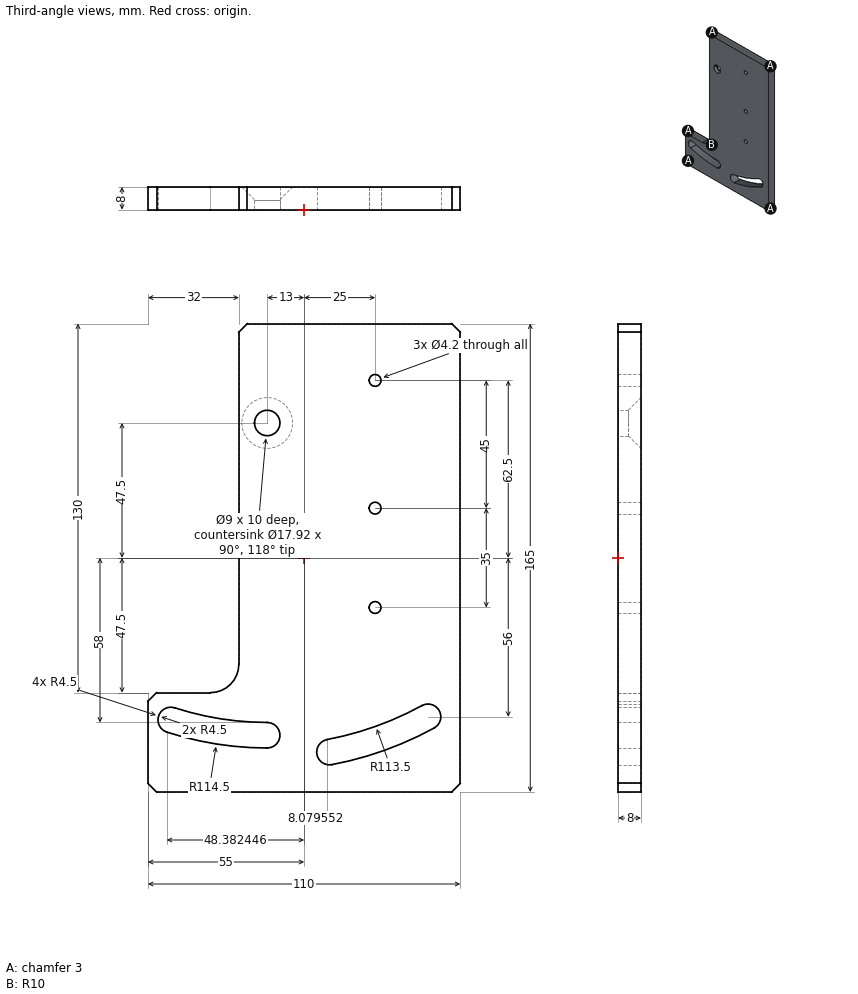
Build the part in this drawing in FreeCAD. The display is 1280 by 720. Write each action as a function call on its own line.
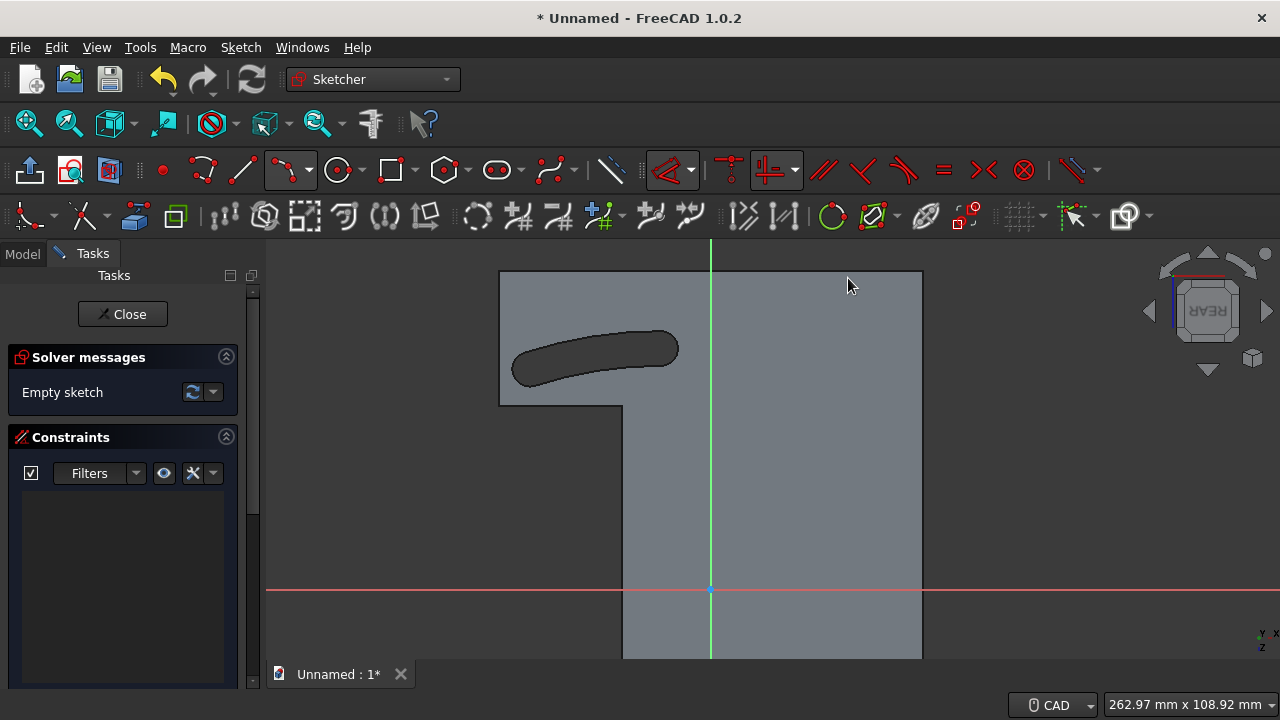
click(284, 170)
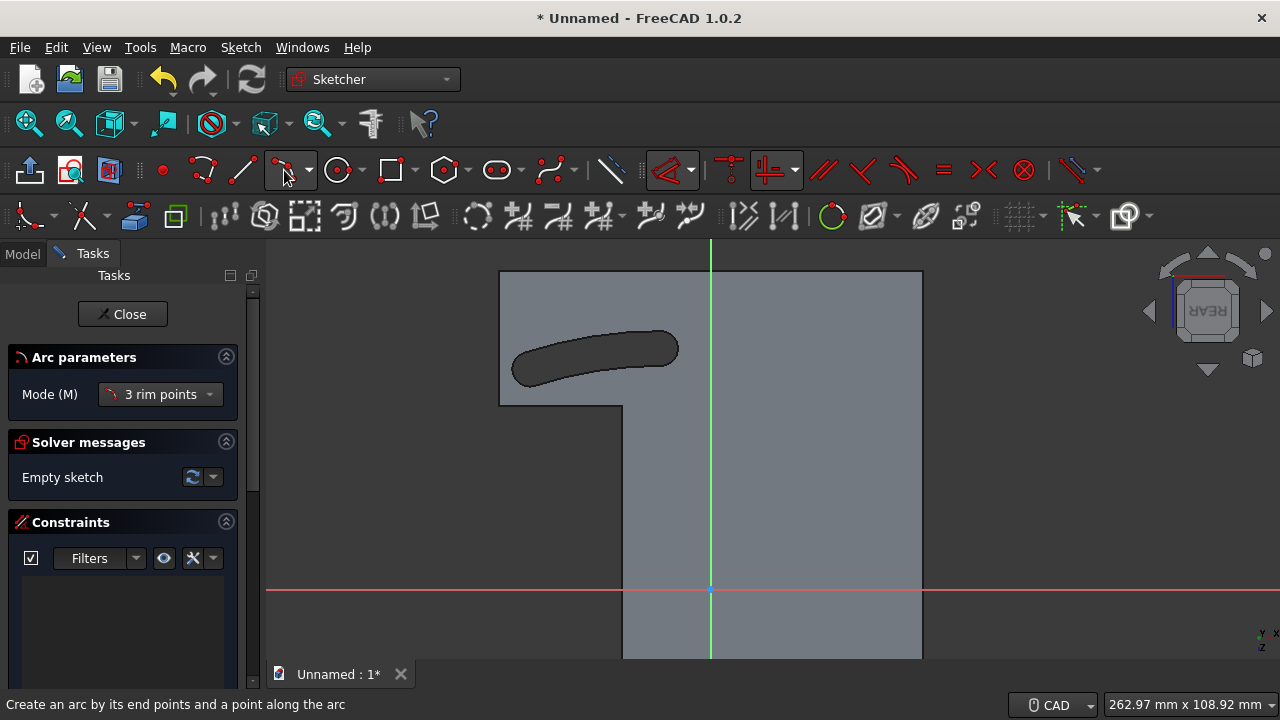
click(661, 366)
click(661, 331)
click(678, 349)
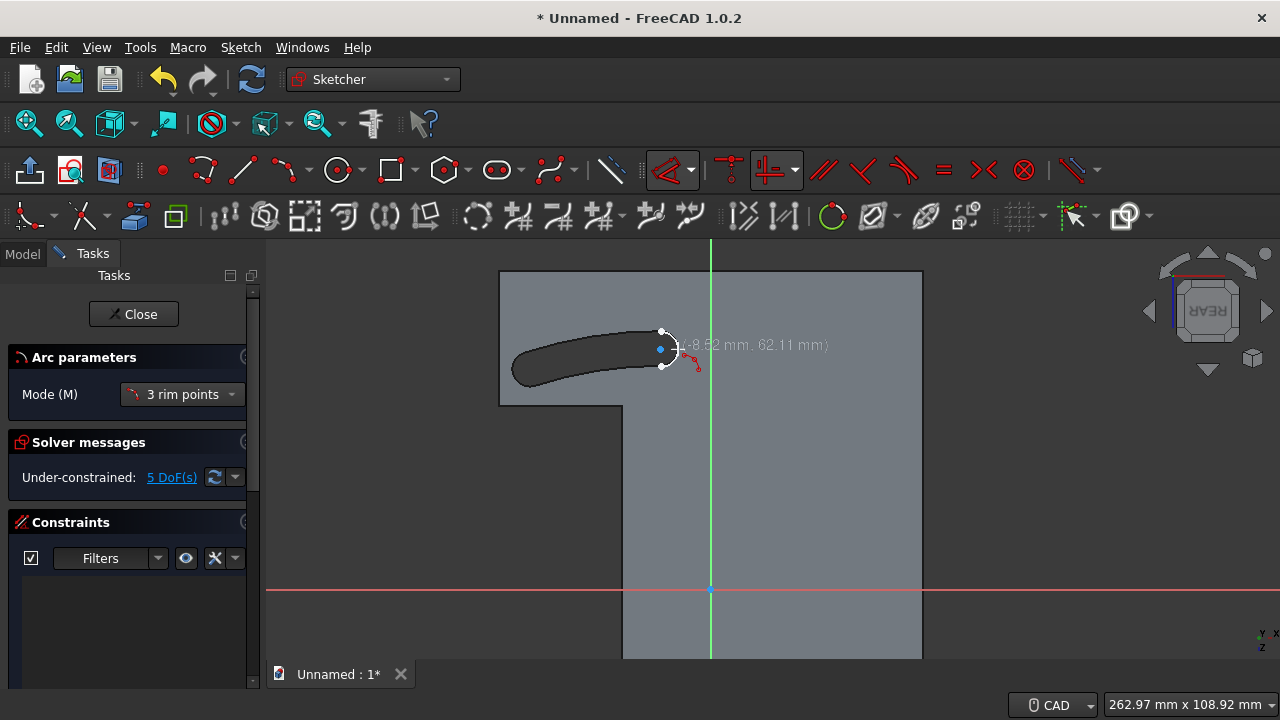
click(661, 332)
click(524, 353)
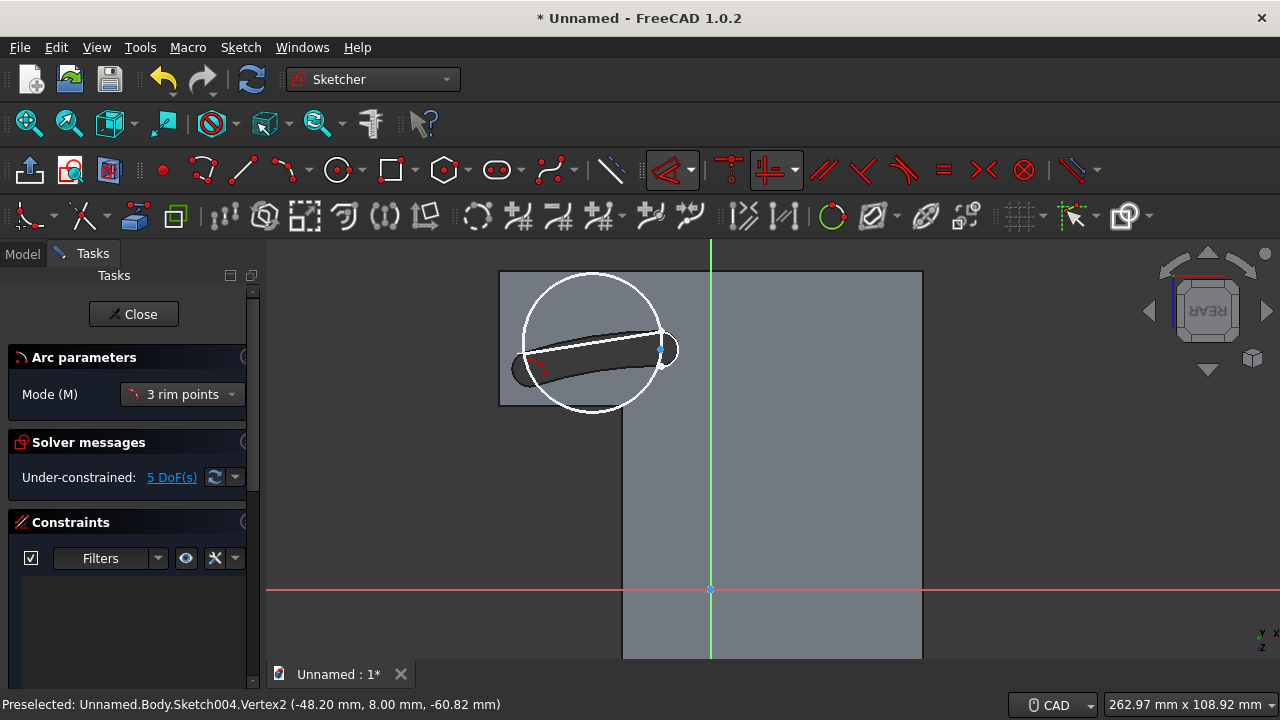
scroll(592, 337, up, 6)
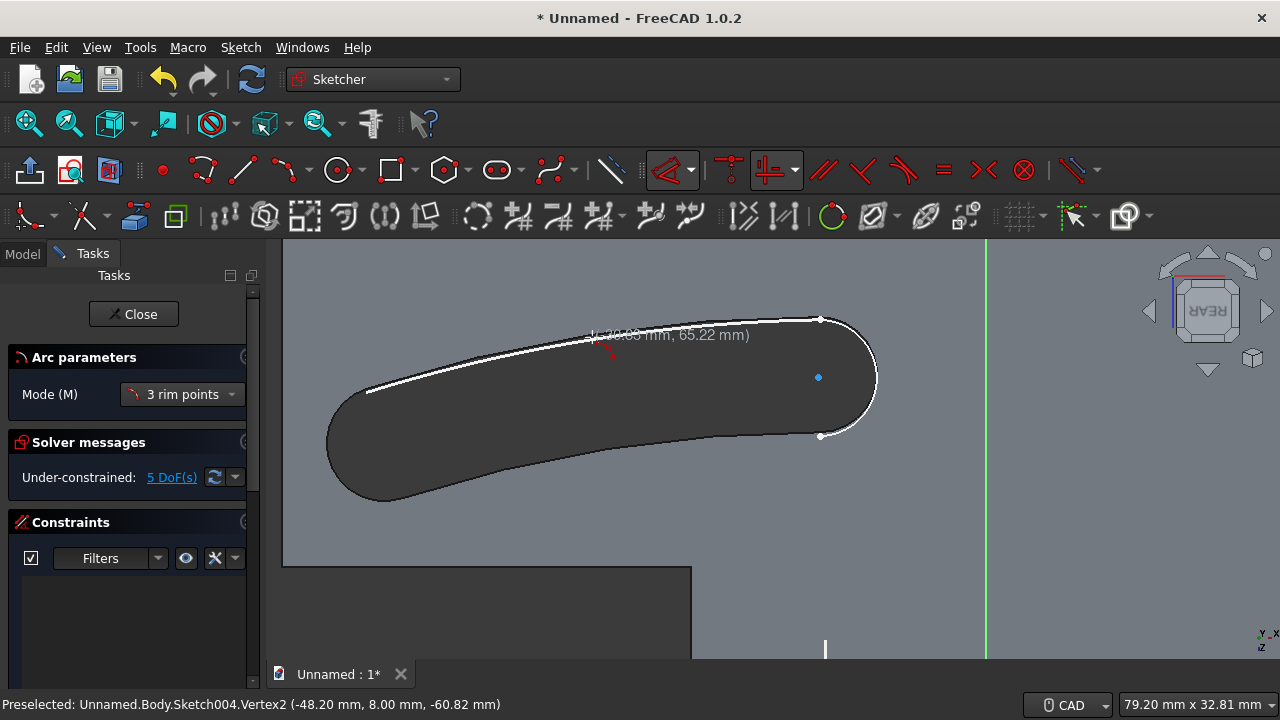
click(590, 335)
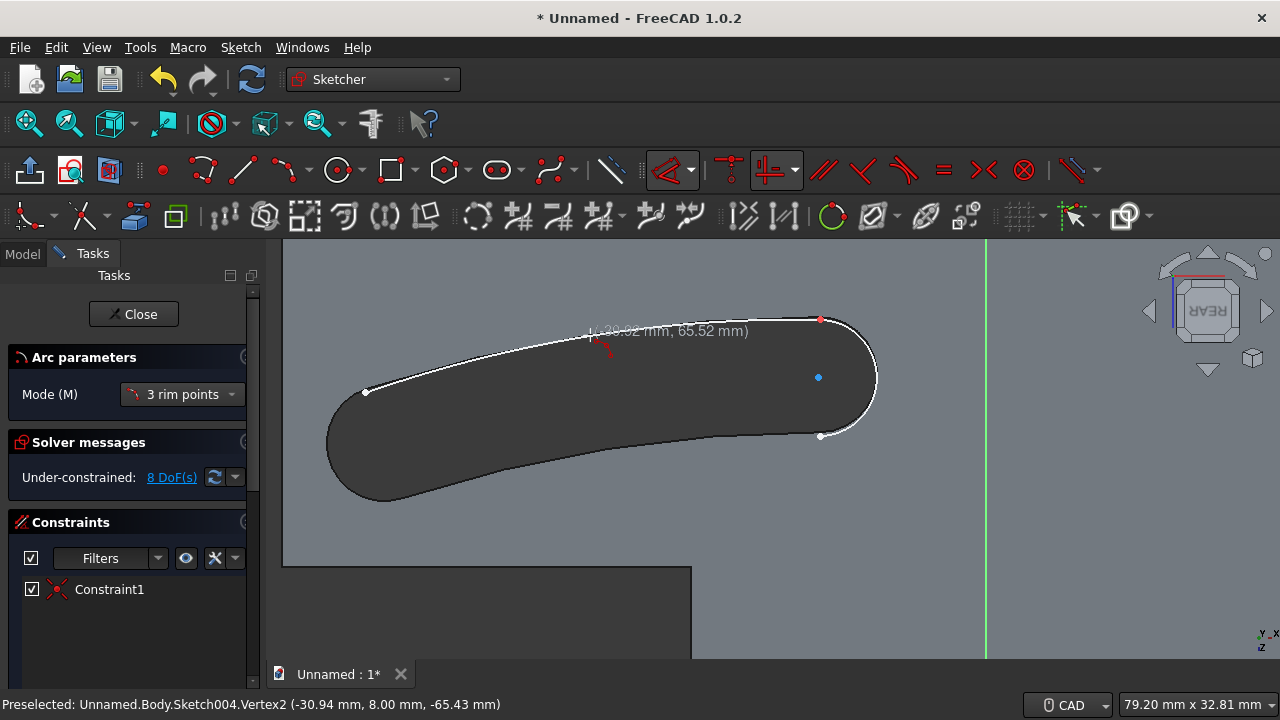
click(365, 393)
click(402, 498)
click(330, 461)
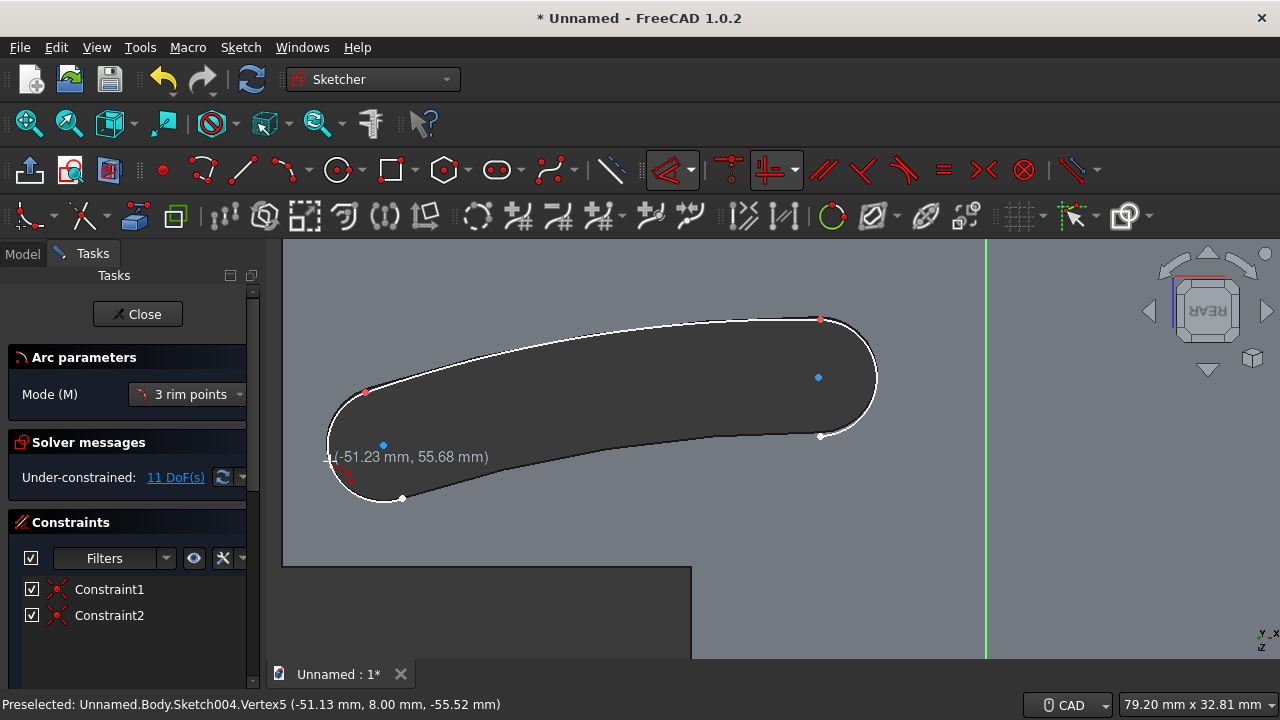
click(402, 499)
click(820, 436)
click(608, 449)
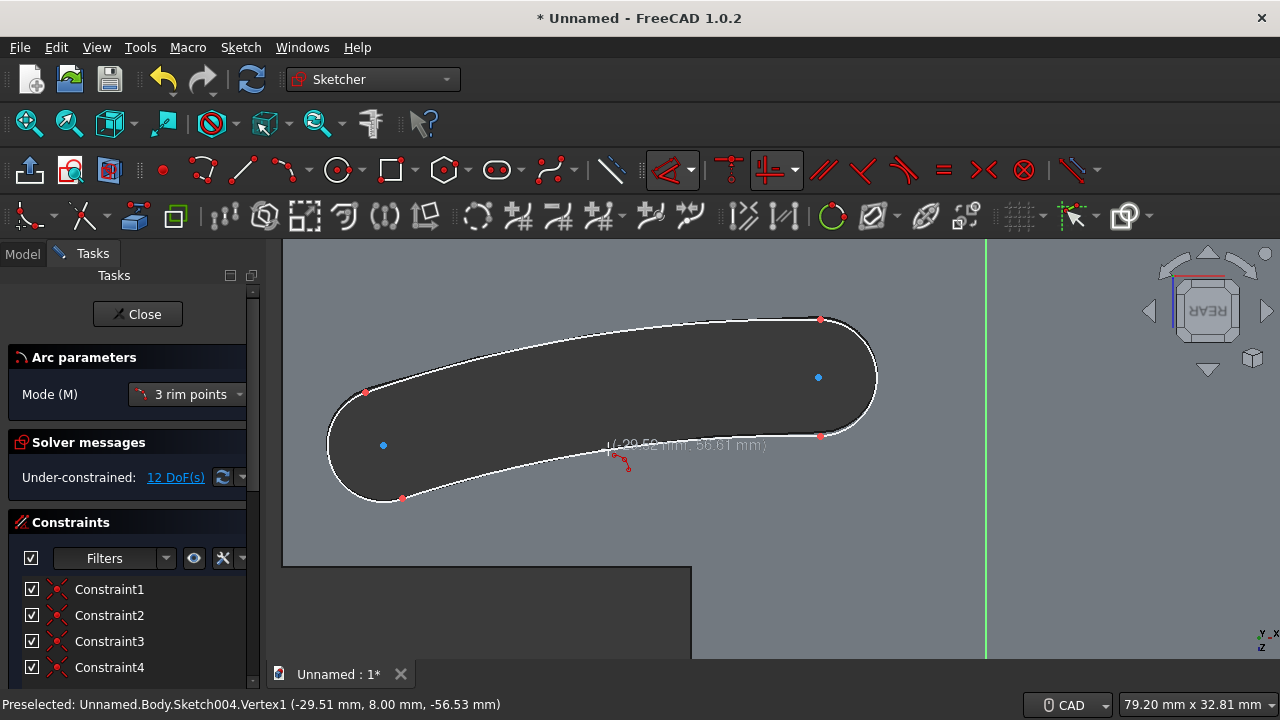
click(1089, 355)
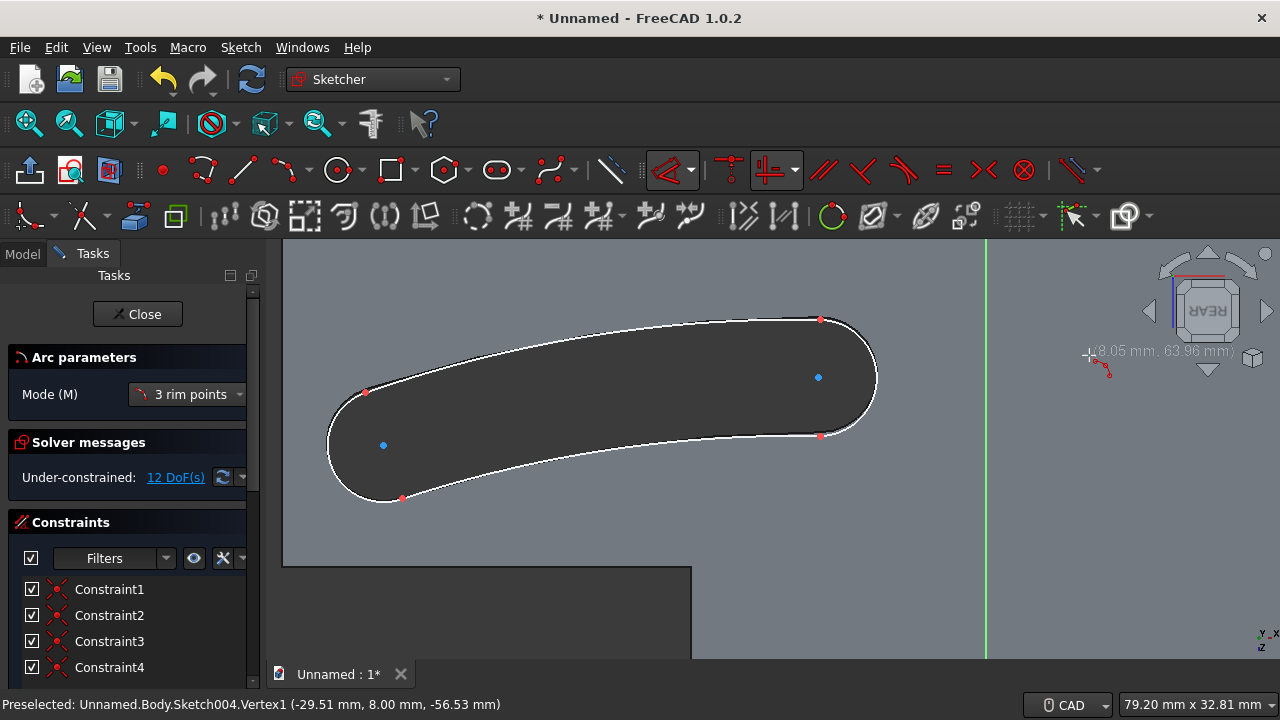
scroll(593, 337, down, 6)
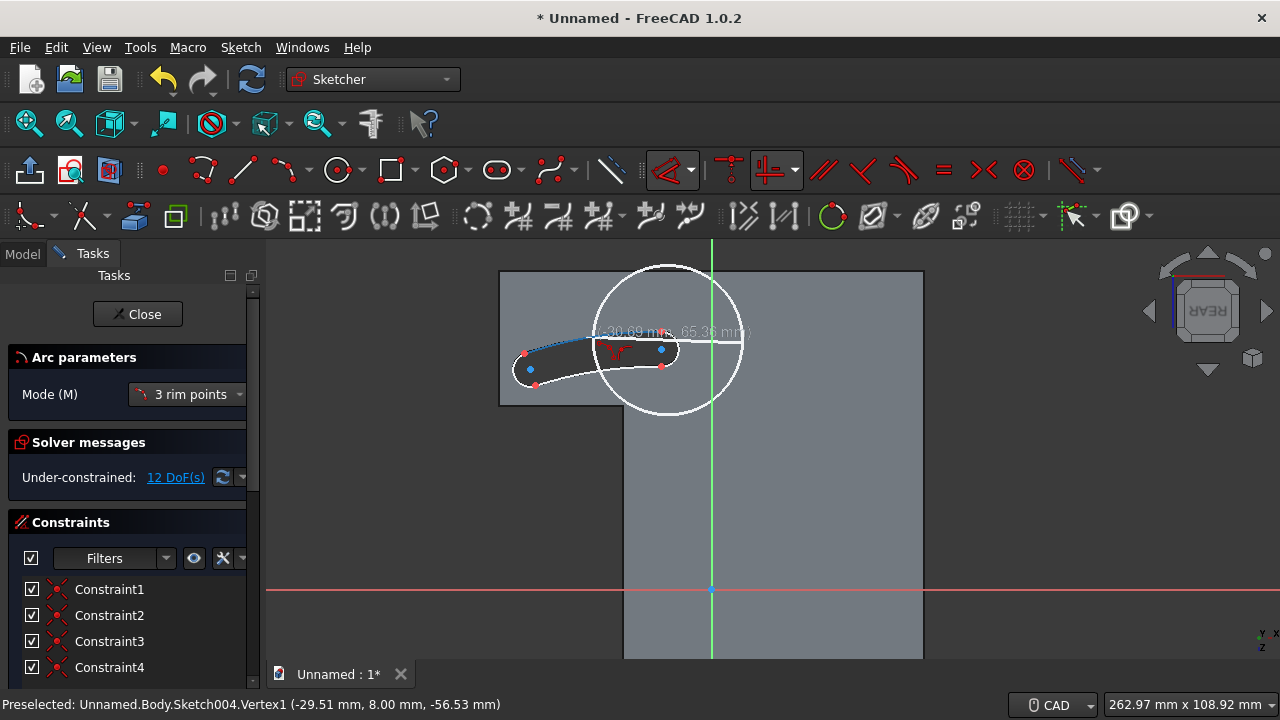
click(872, 389)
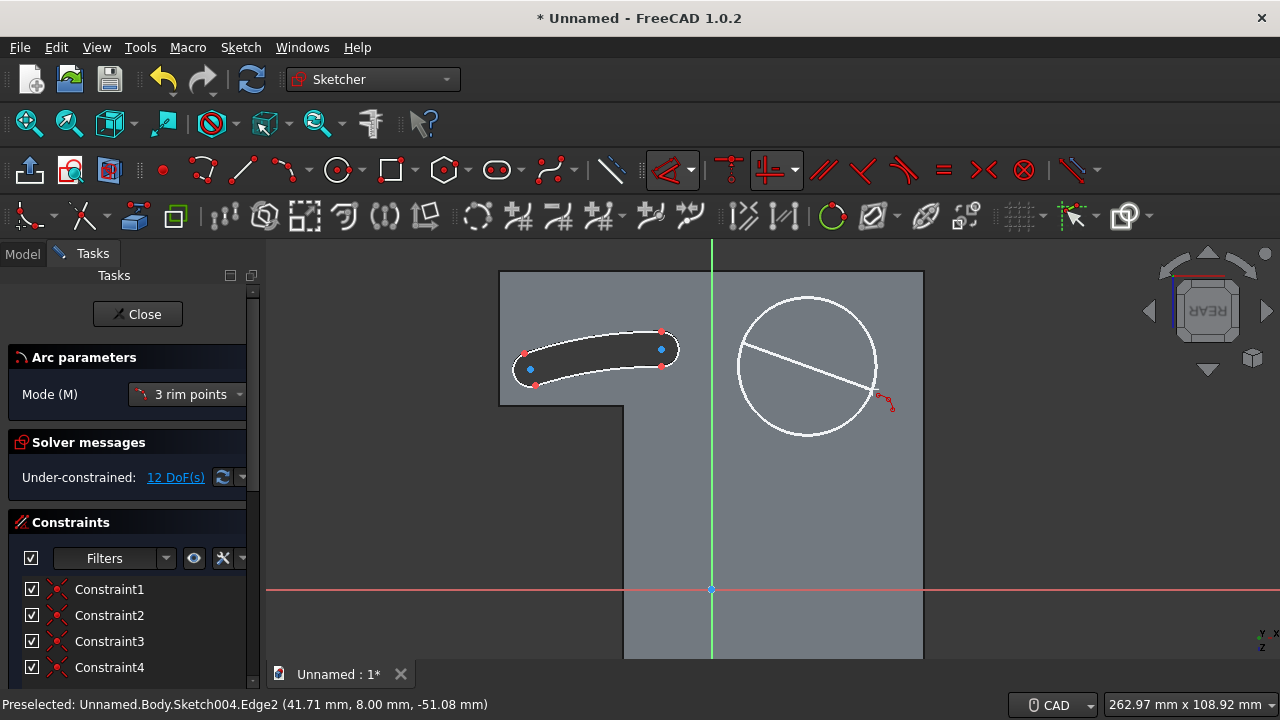
scroll(809, 361, up, 6)